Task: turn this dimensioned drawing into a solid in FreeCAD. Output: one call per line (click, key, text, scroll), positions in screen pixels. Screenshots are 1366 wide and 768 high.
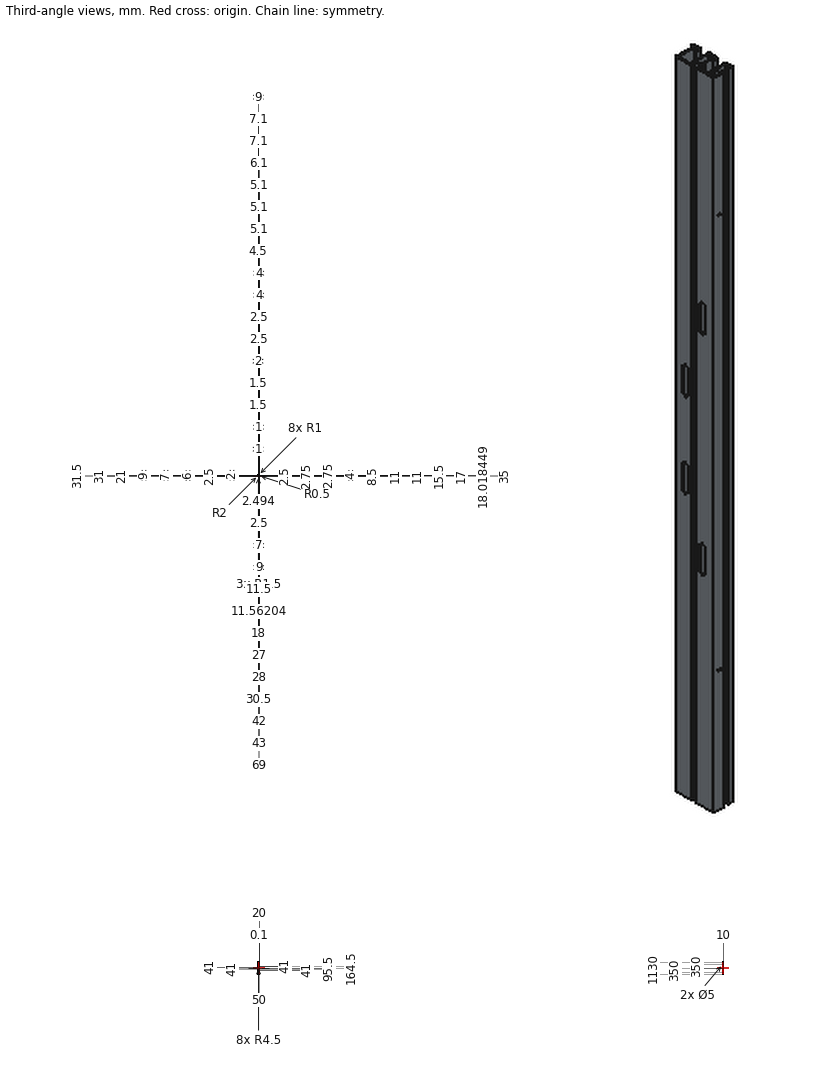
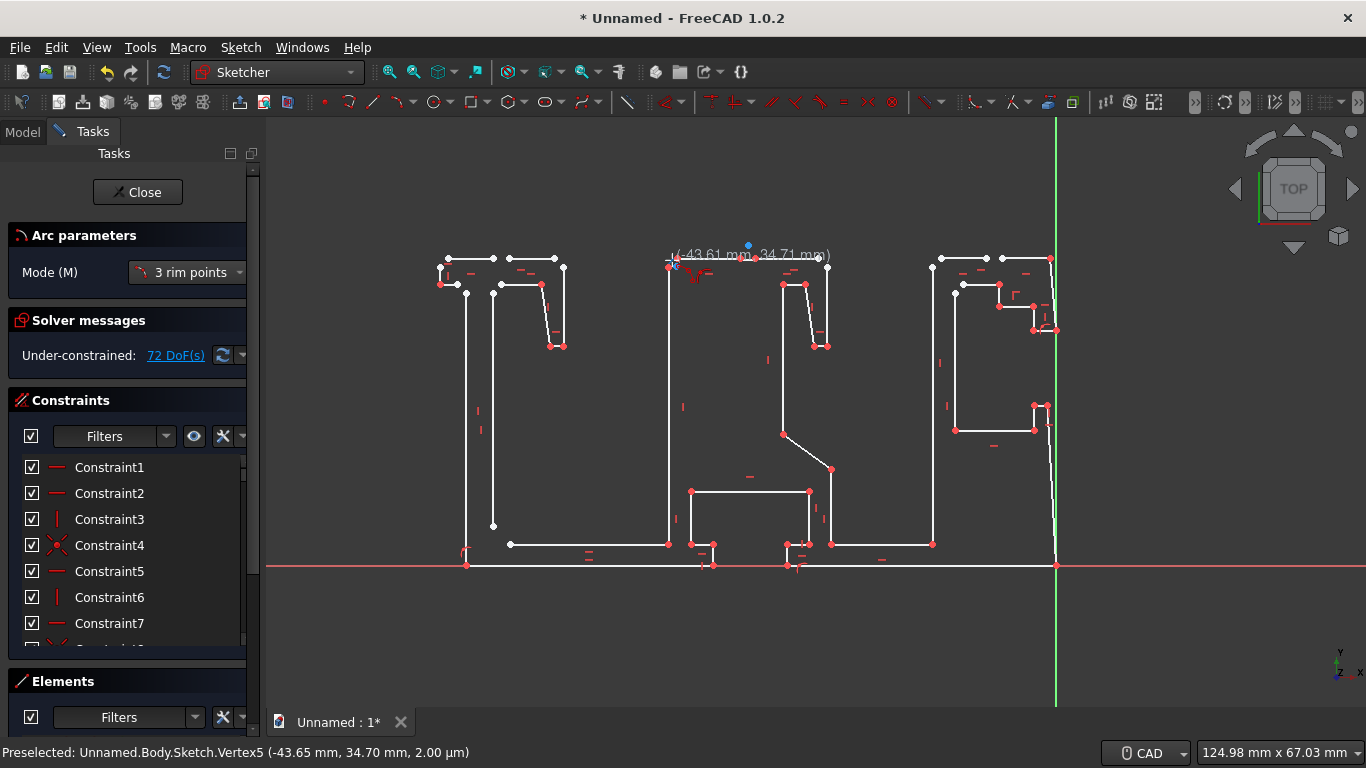
click(511, 545)
click(493, 527)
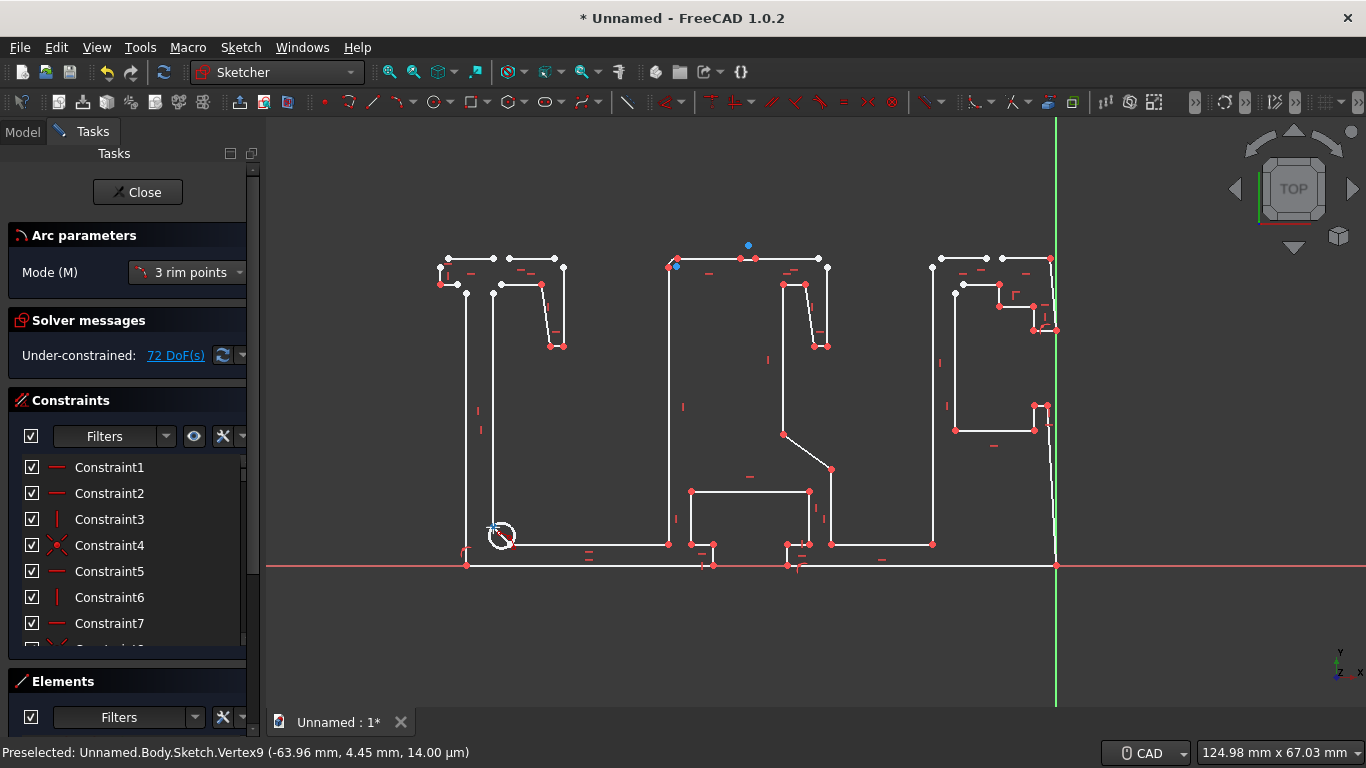
scroll(498, 539, up, 6)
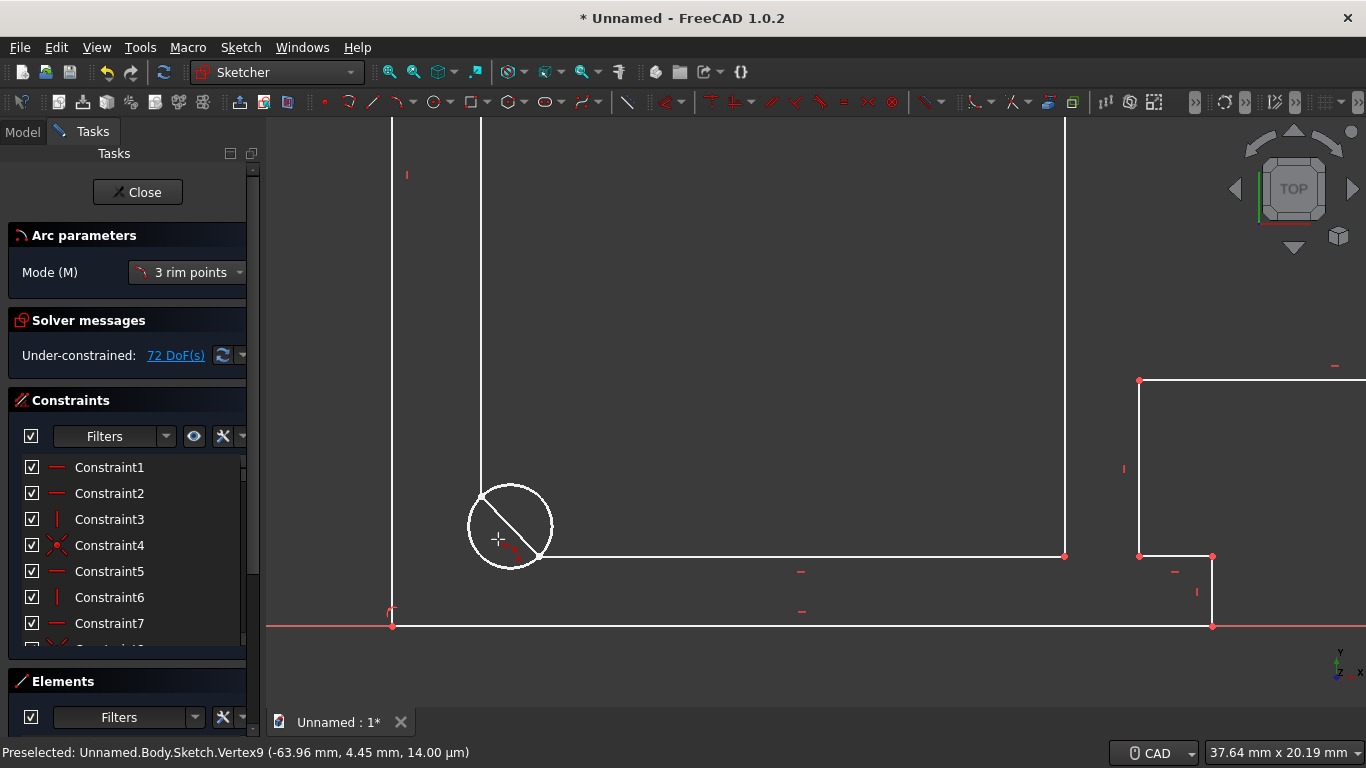
click(498, 536)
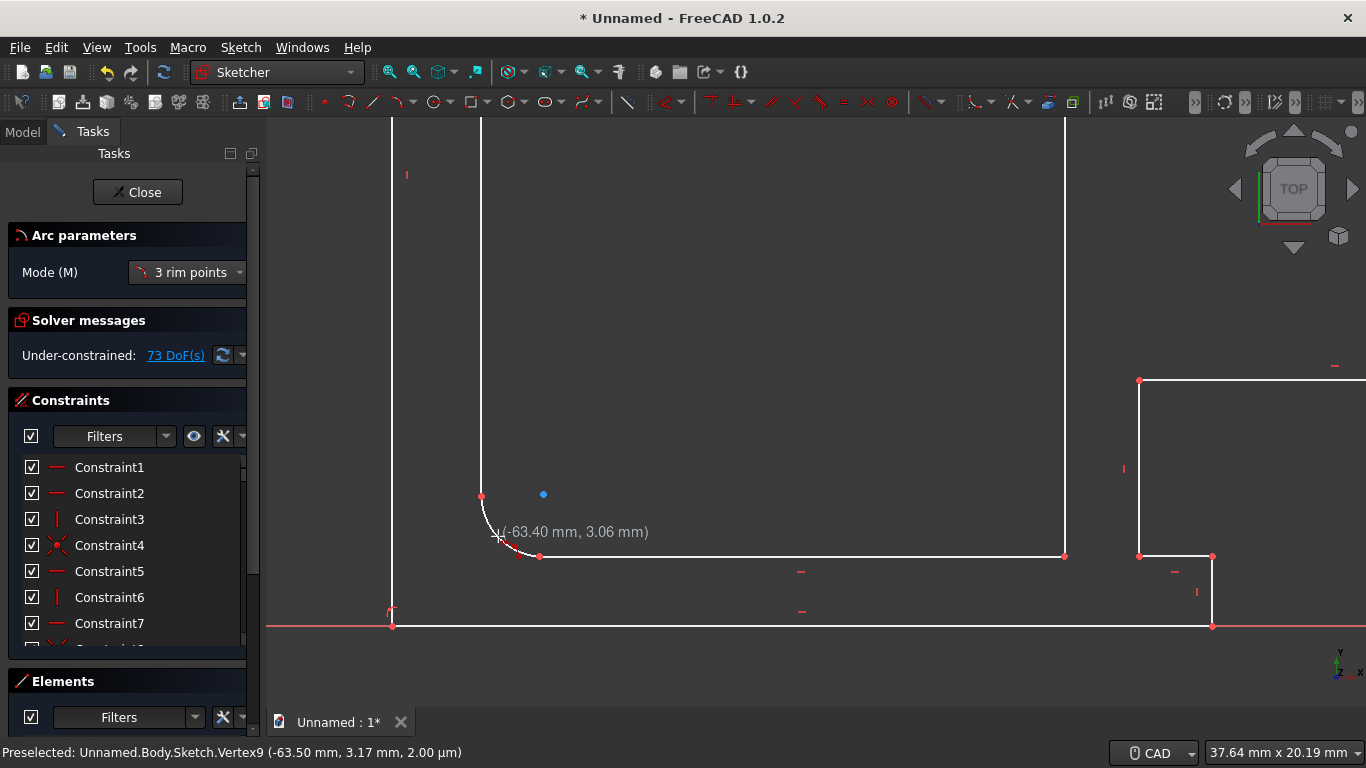
scroll(497, 540, down, 6)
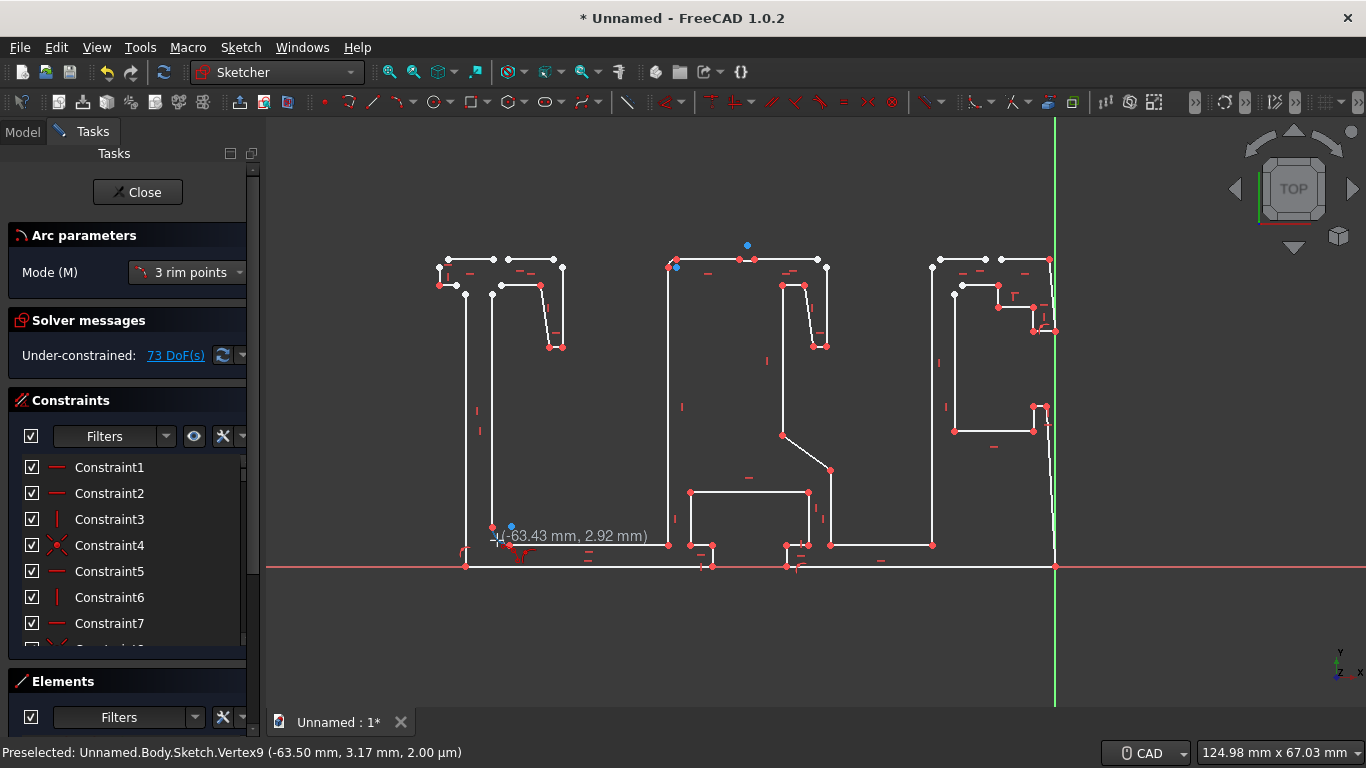
scroll(492, 294, up, 2)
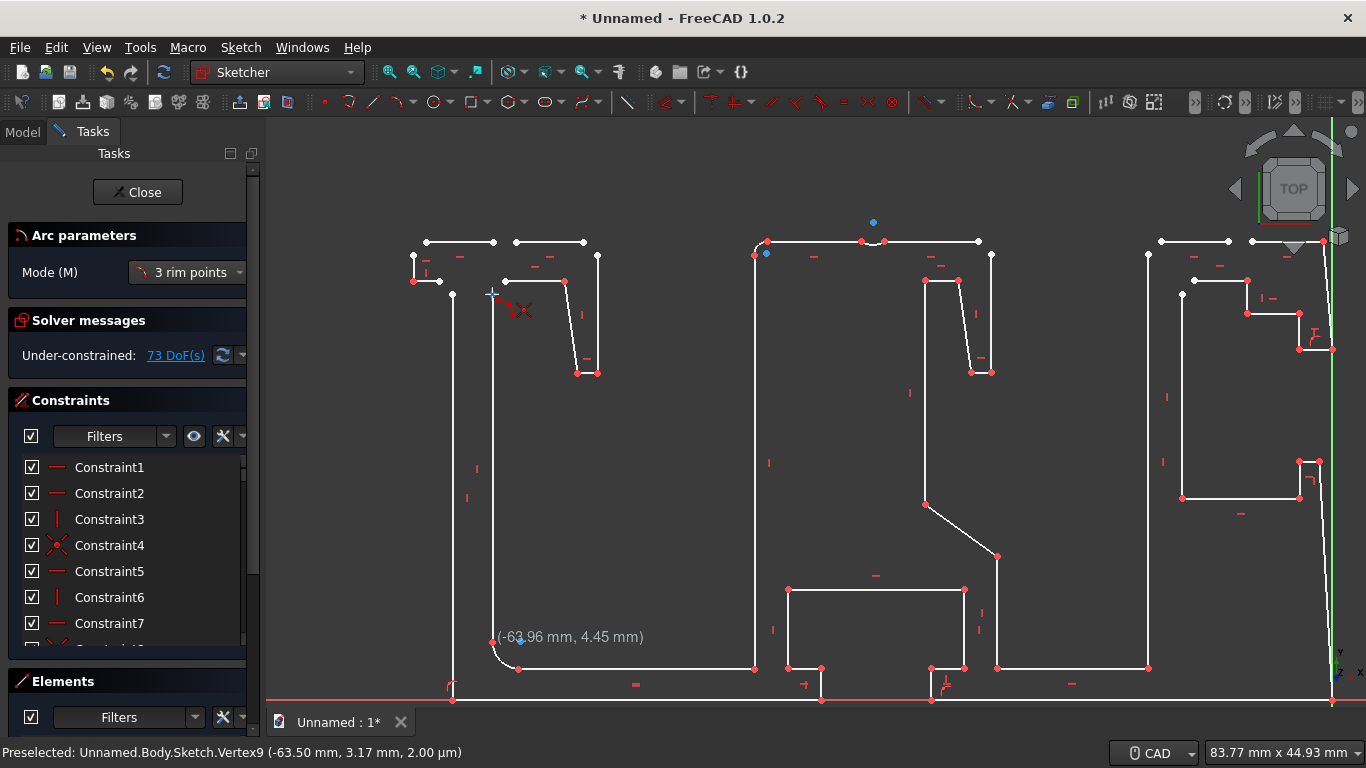
click(493, 294)
click(506, 281)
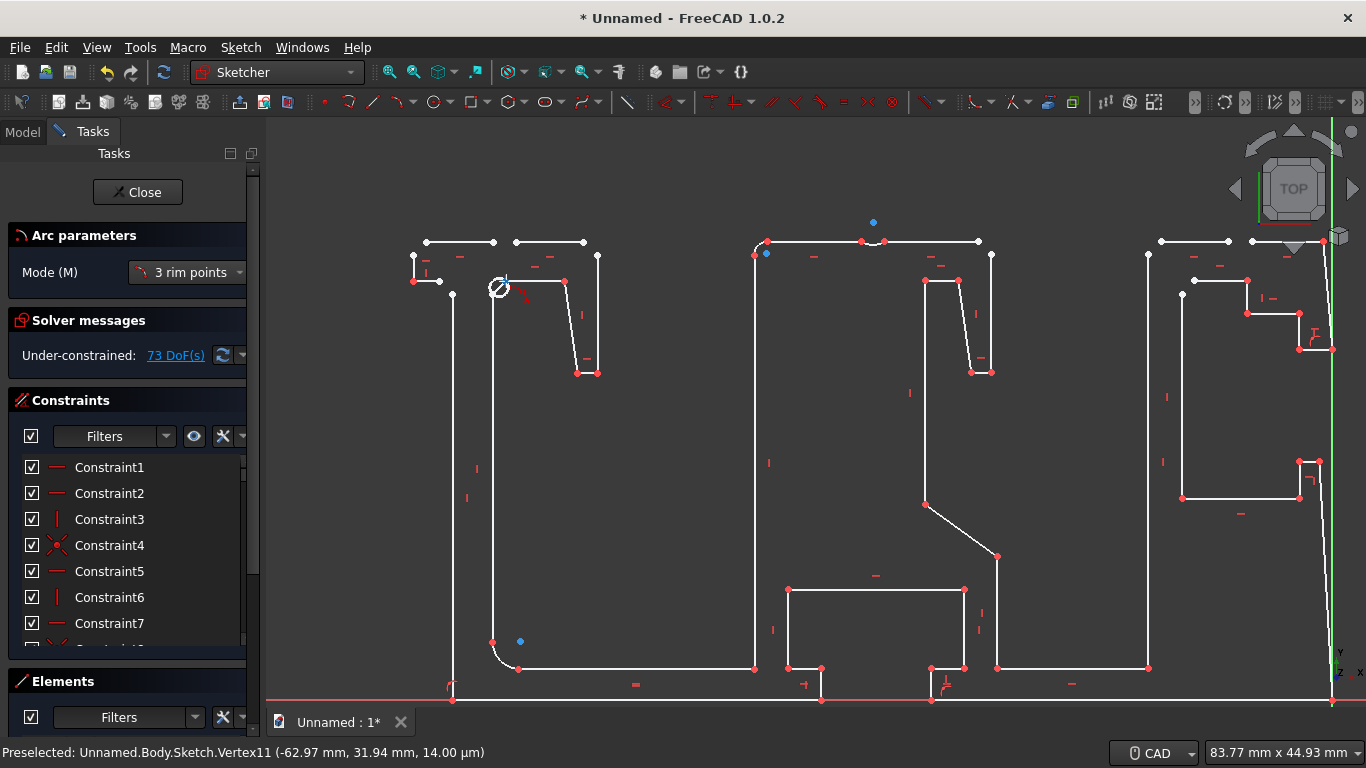
scroll(496, 284, up, 8)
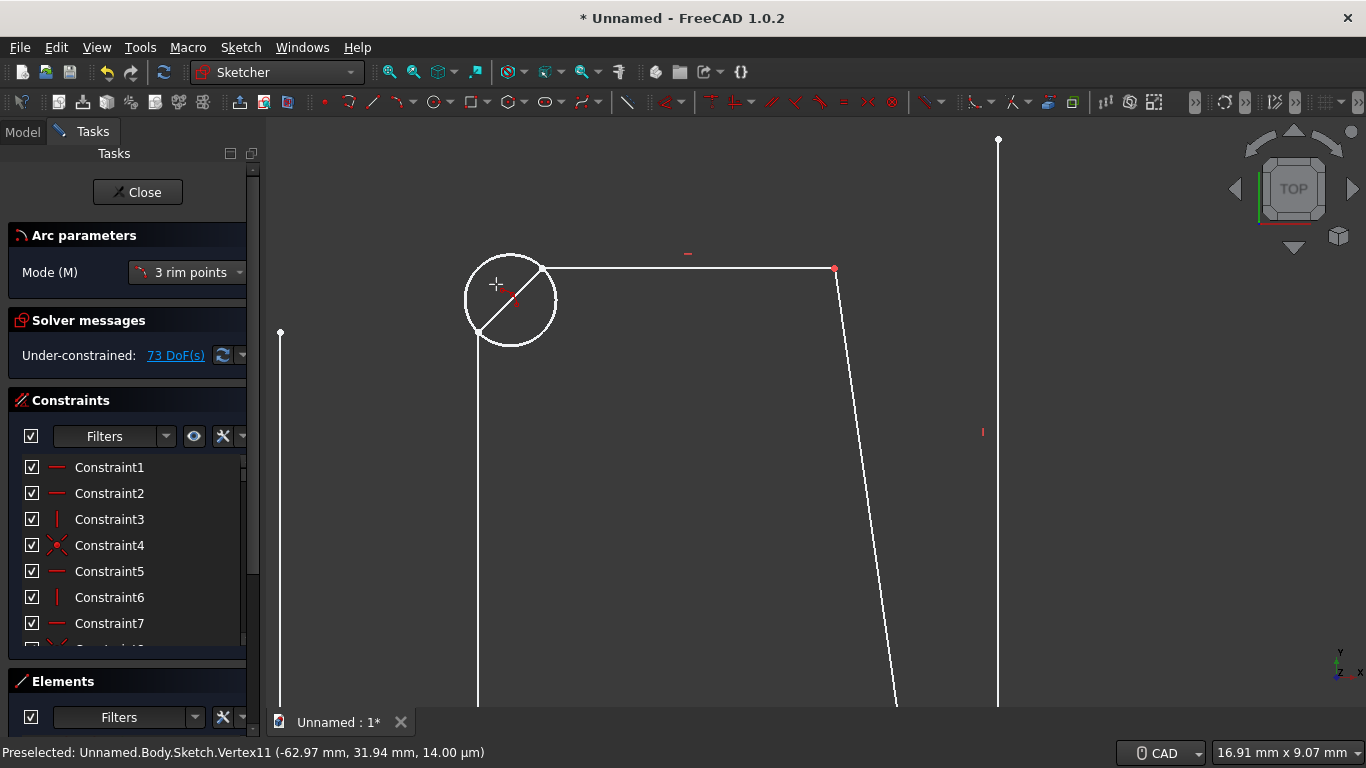
click(495, 283)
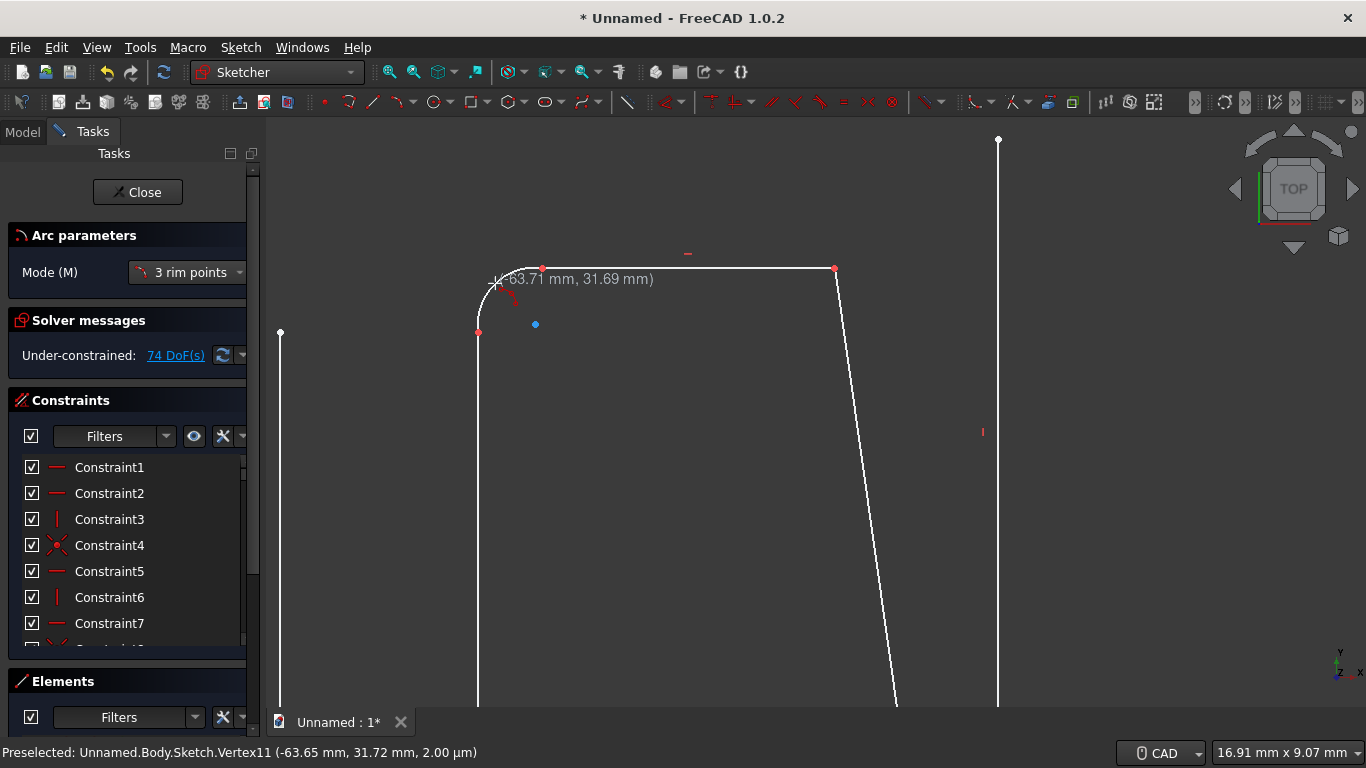
scroll(495, 288, down, 10)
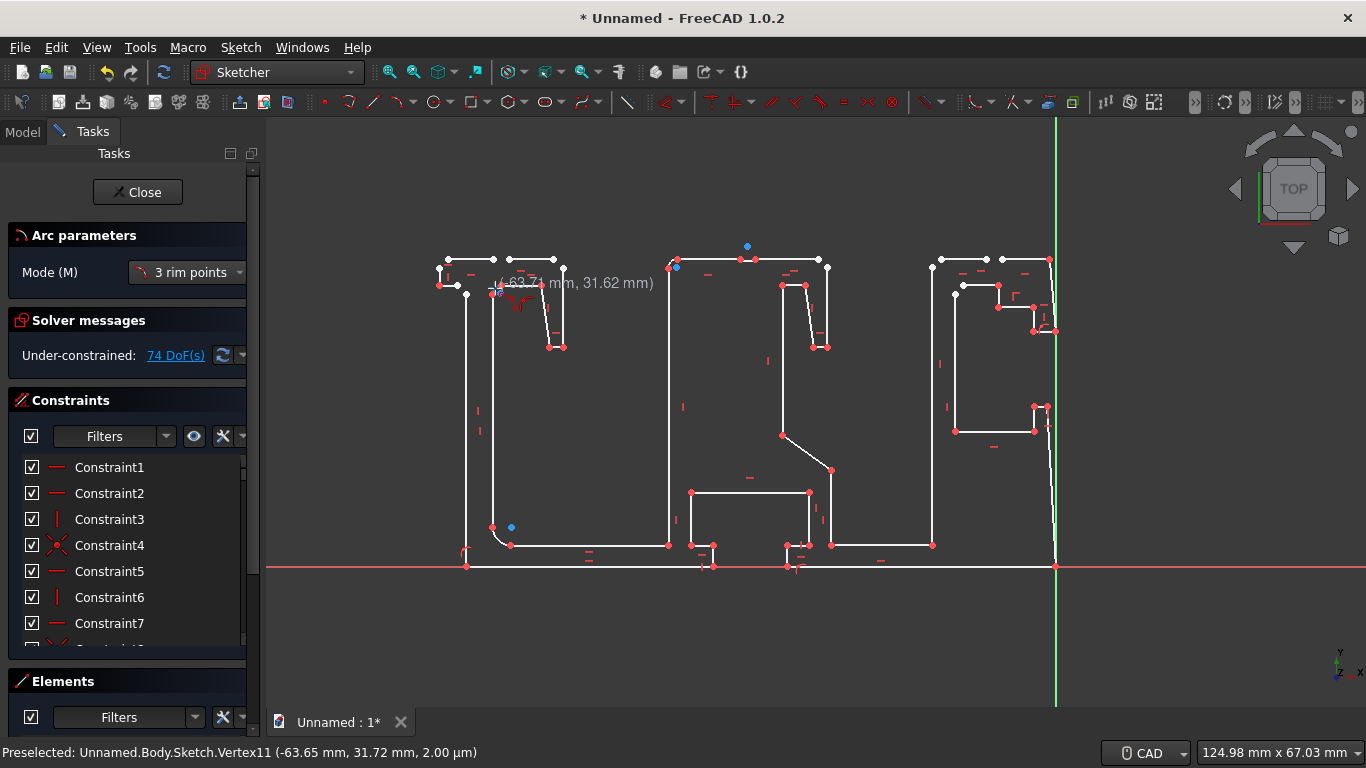
scroll(563, 267, up, 2)